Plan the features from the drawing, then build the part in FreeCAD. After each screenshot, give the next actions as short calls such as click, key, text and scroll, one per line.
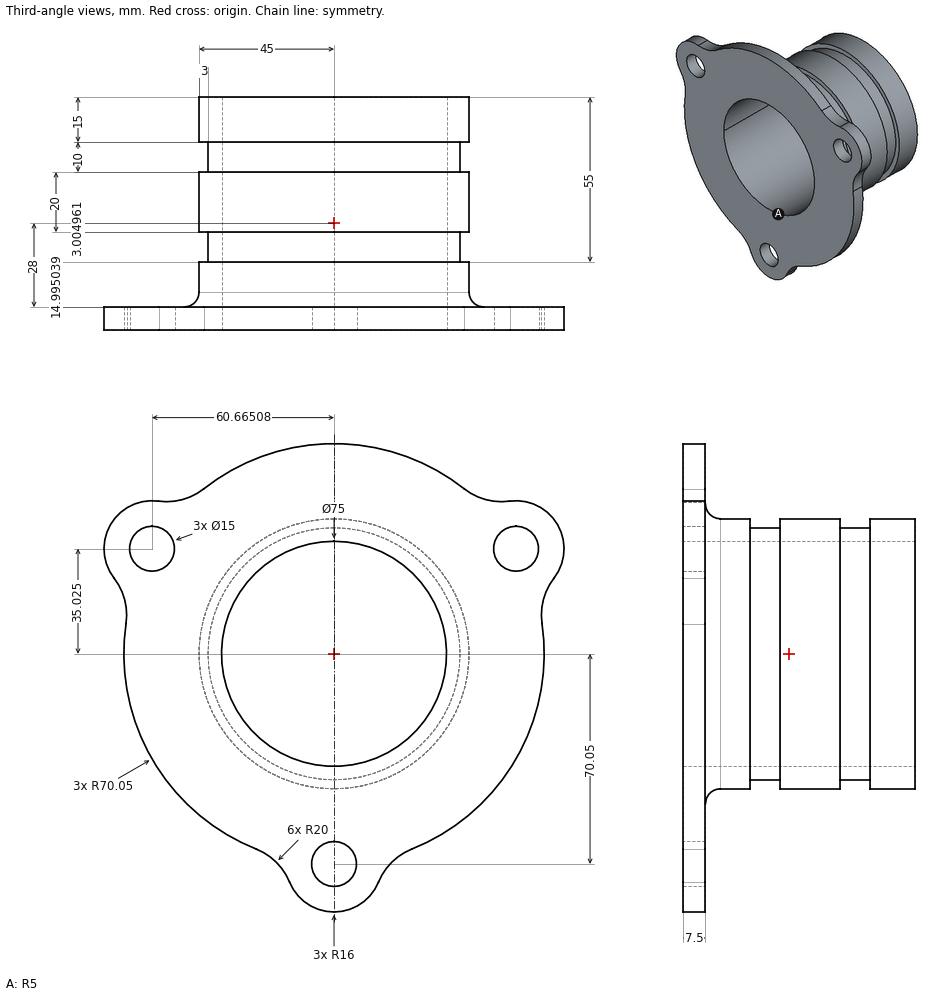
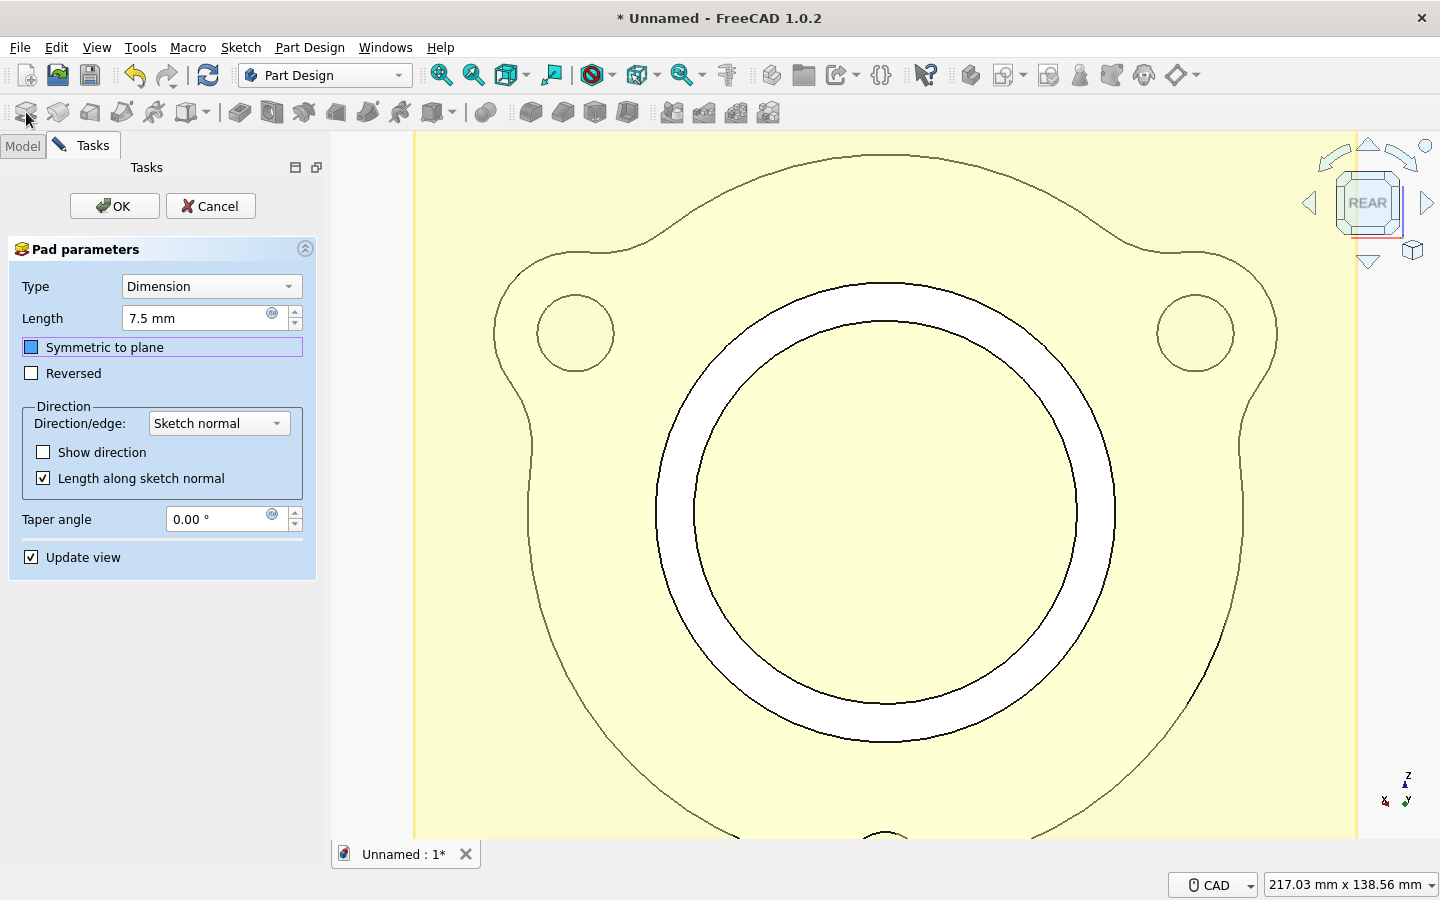
click(115, 206)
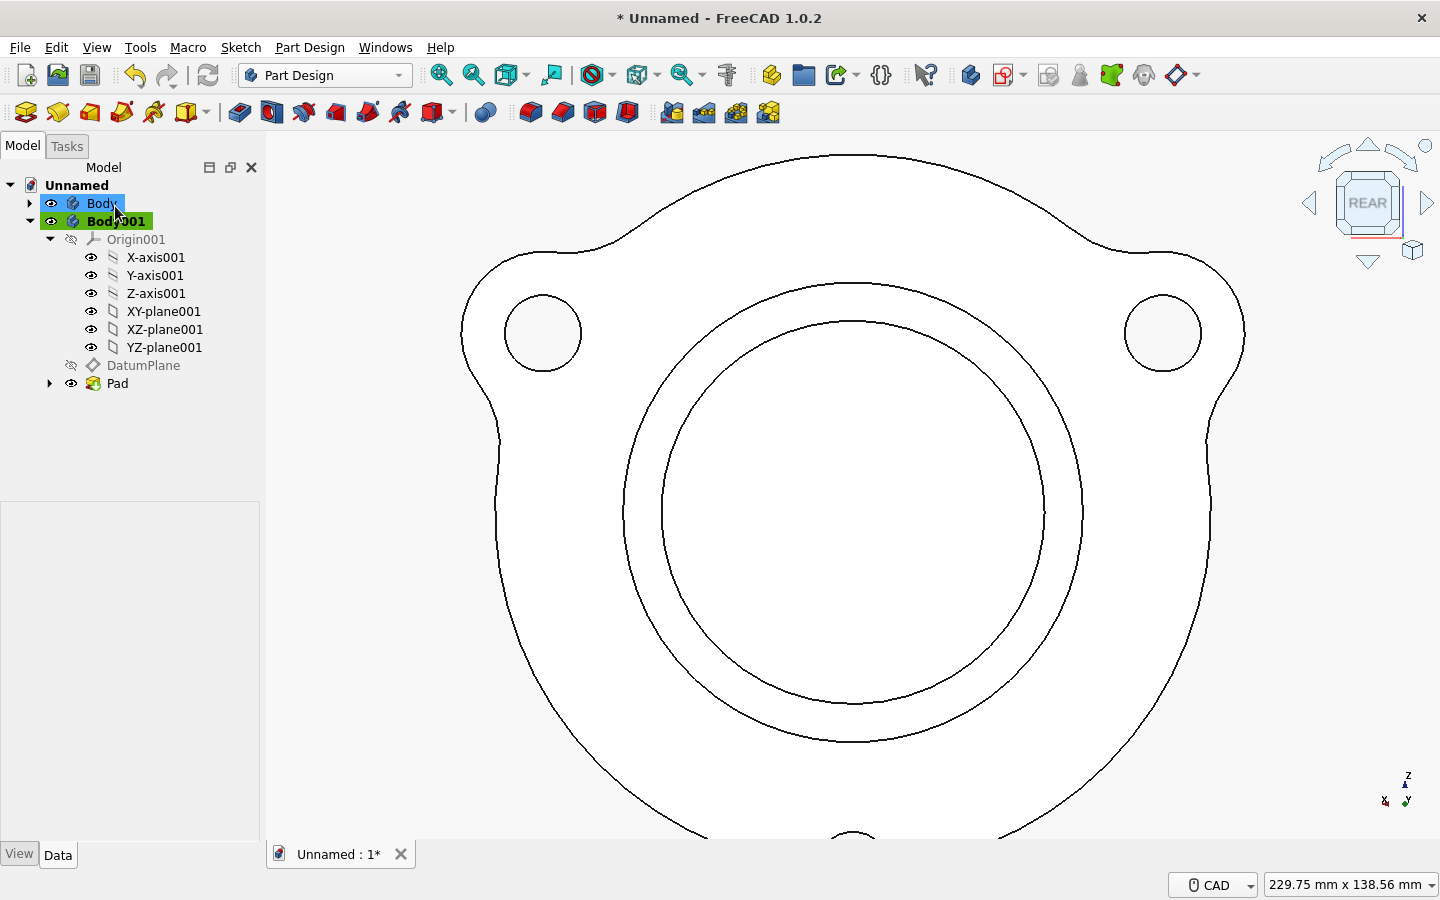
click(442, 76)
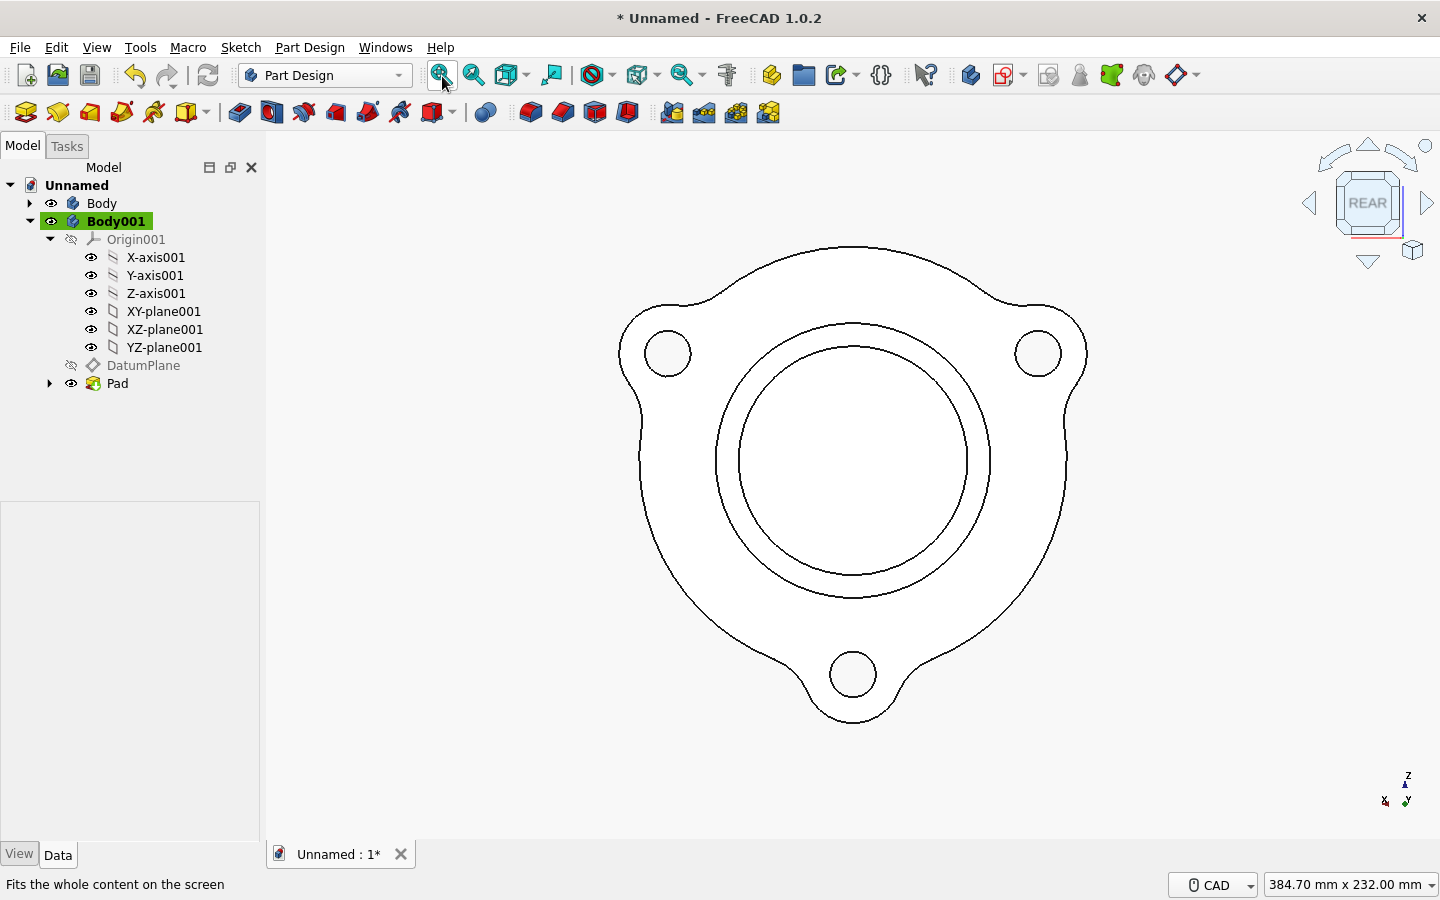
double_click(96, 203)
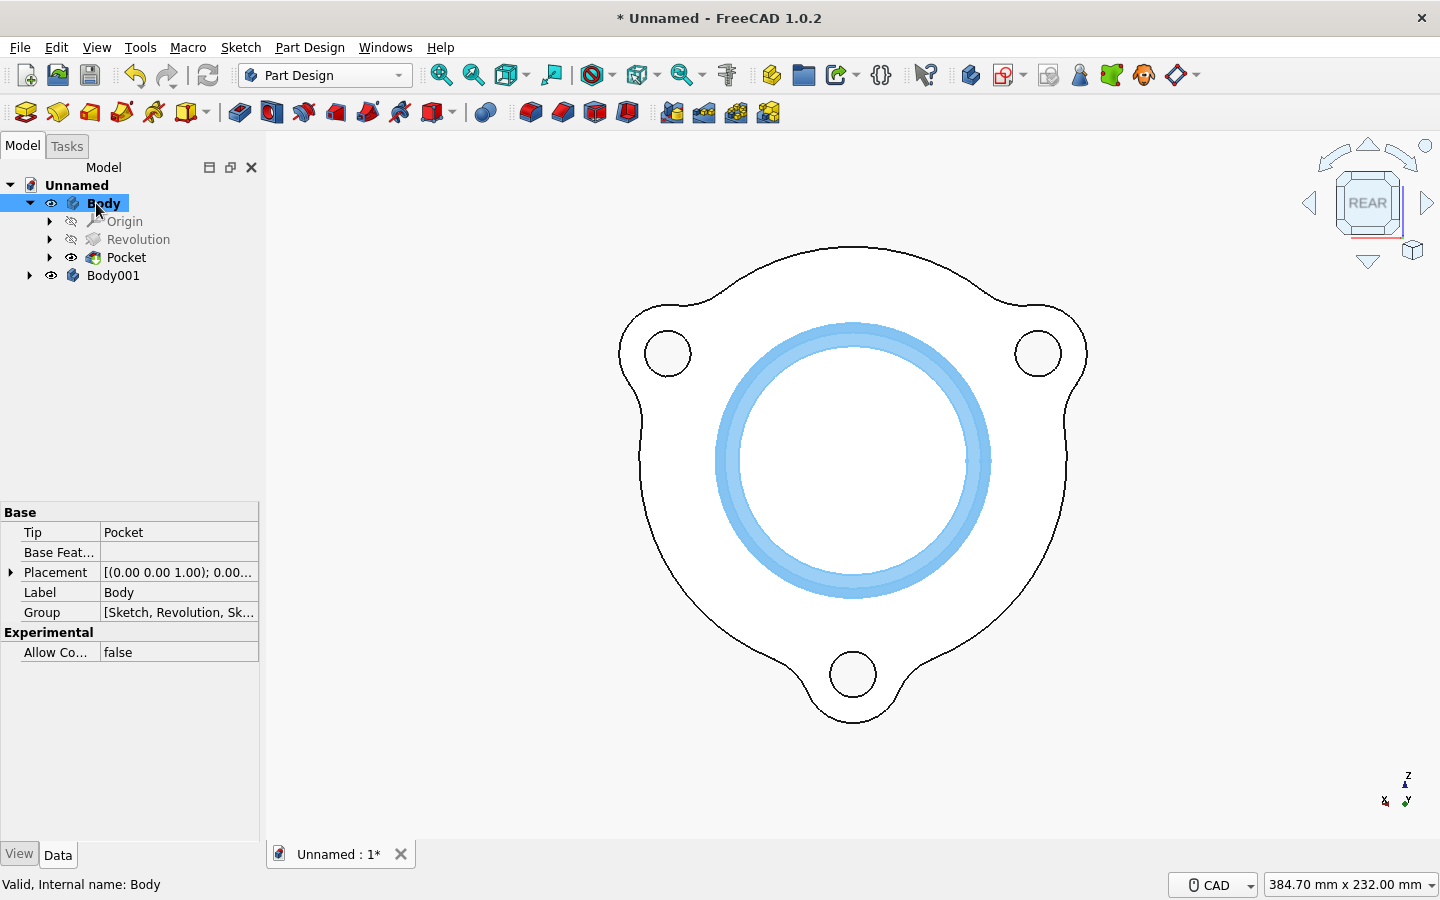
click(96, 203)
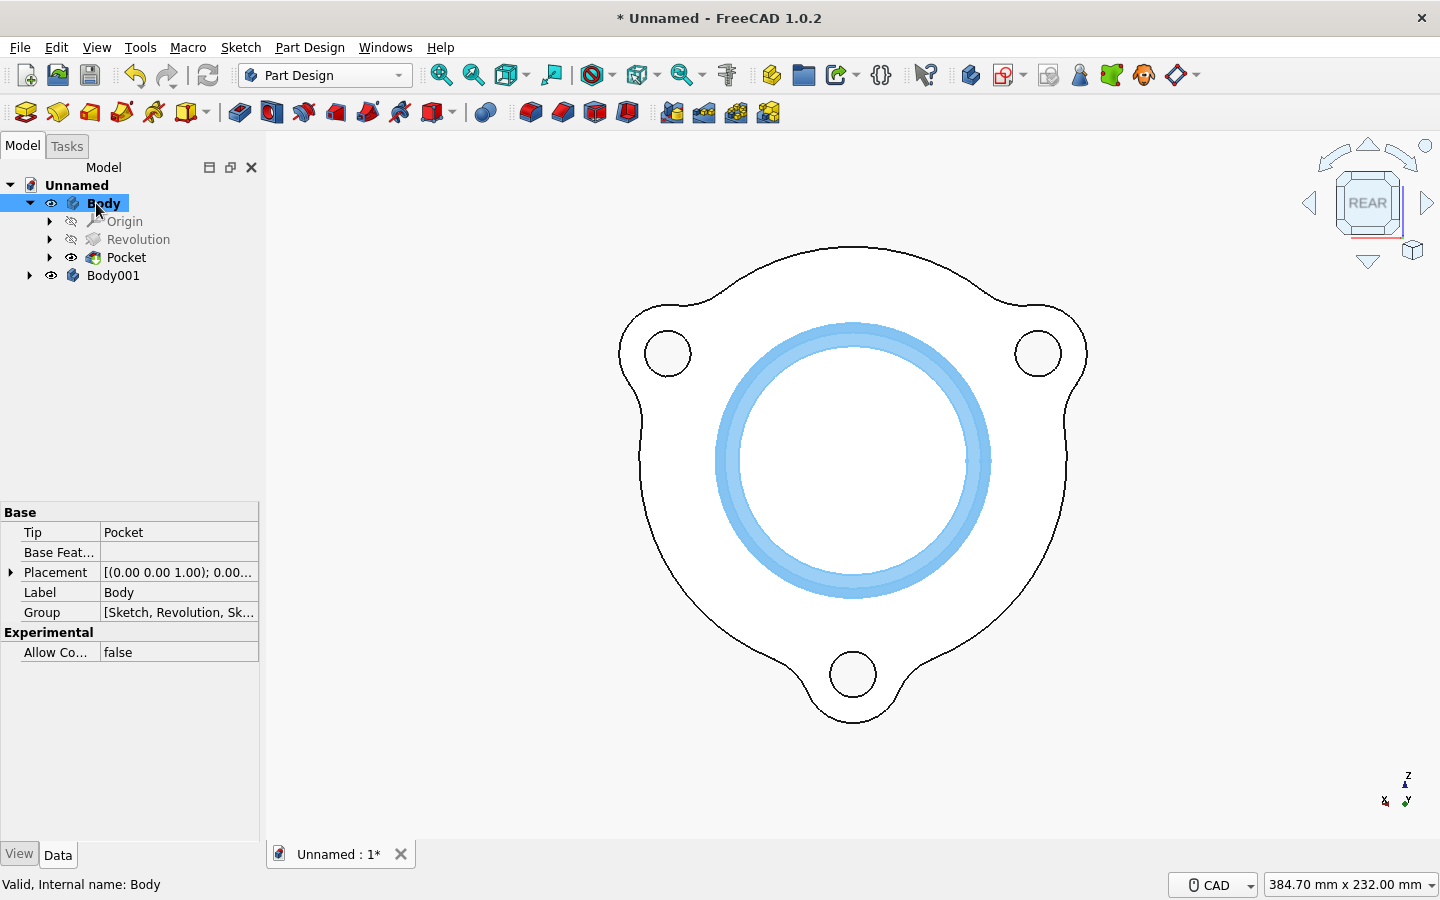
click(146, 652)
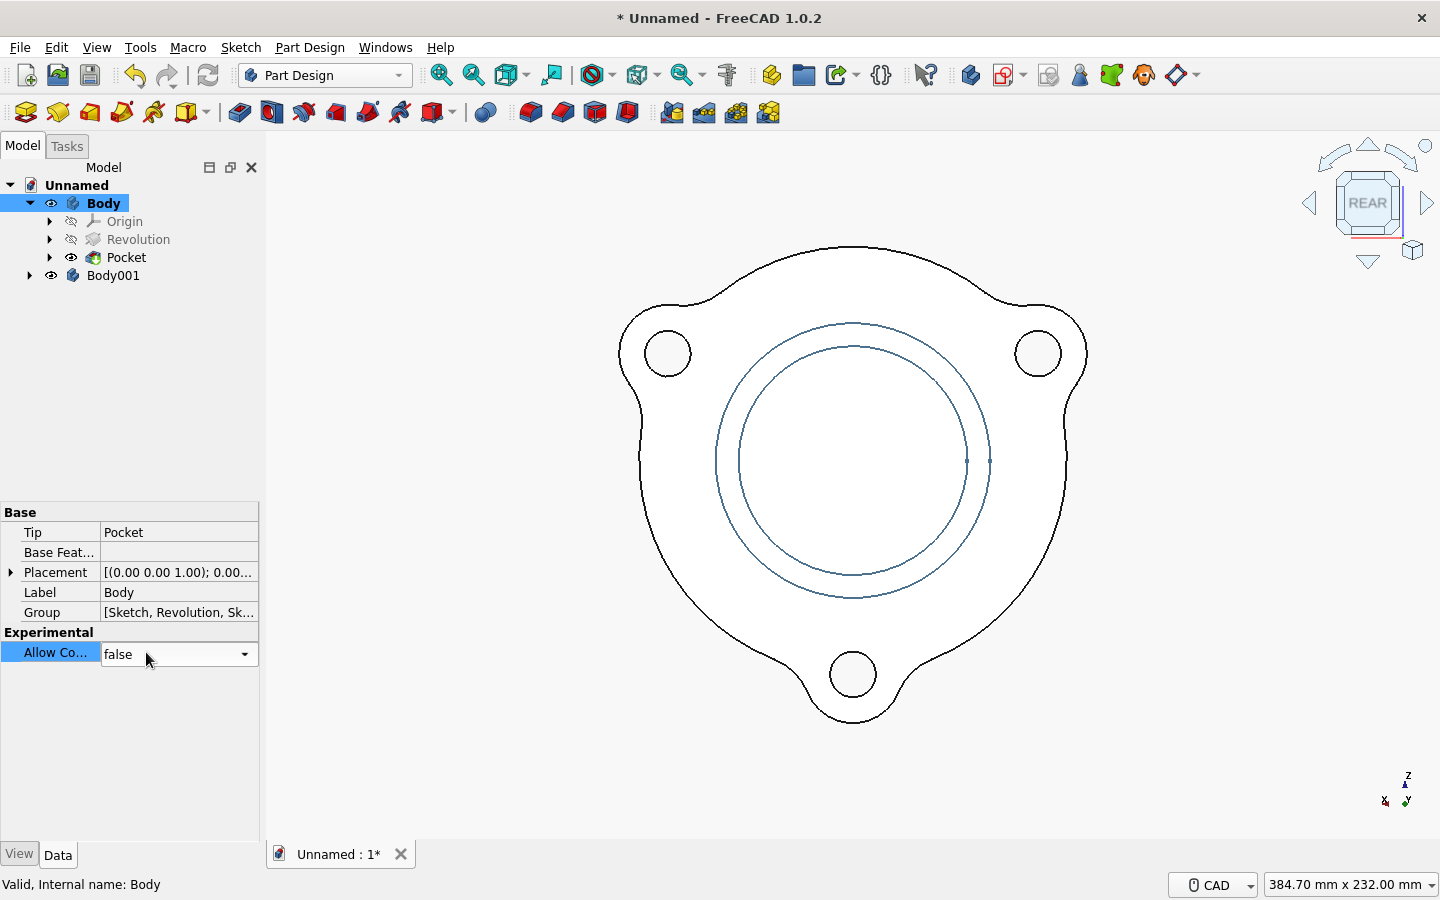
click(146, 652)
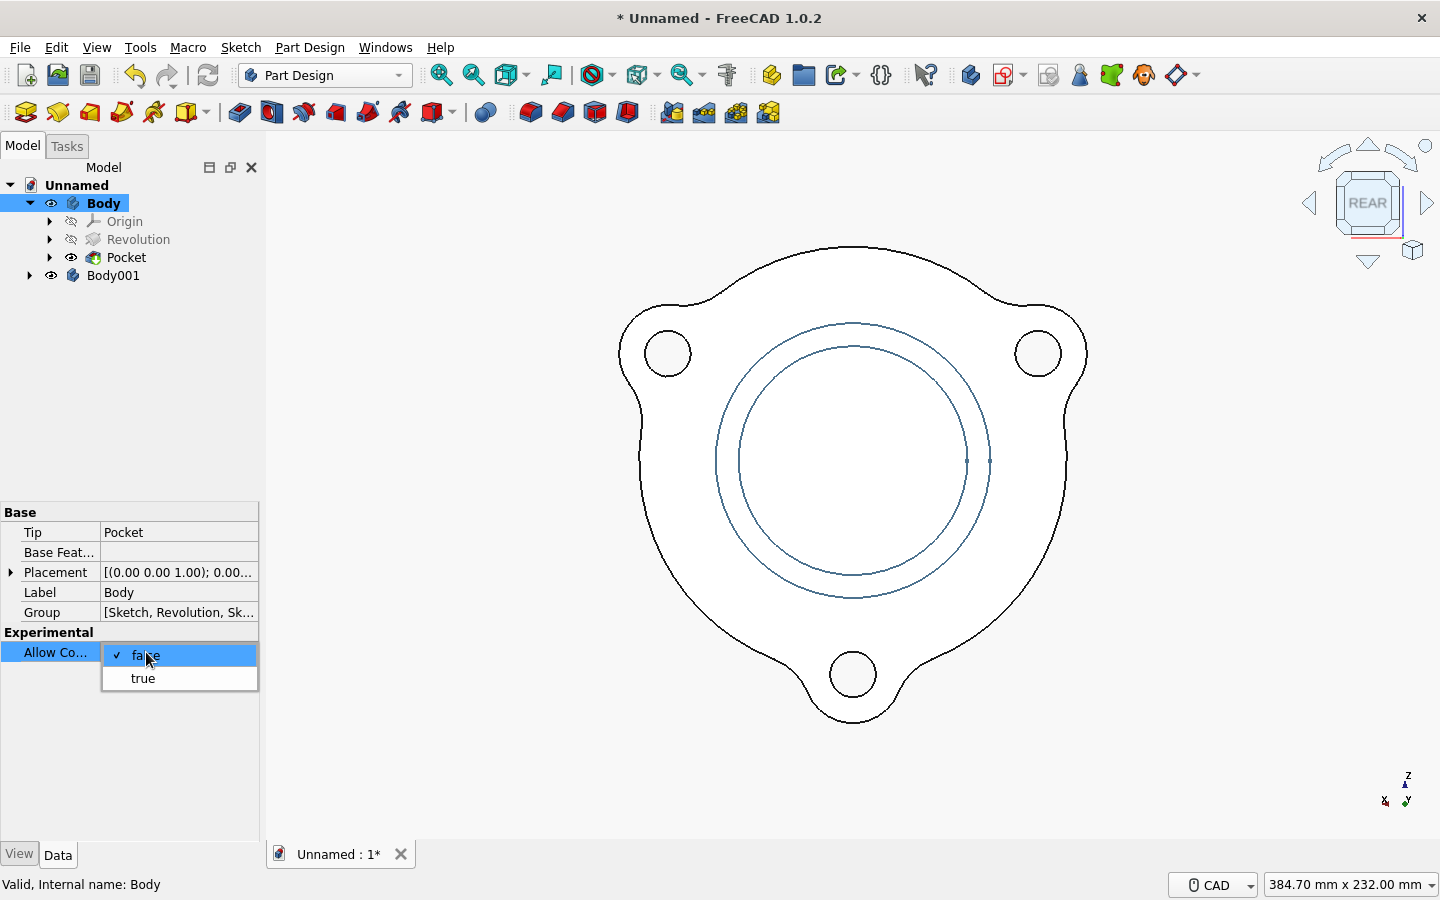
click(179, 678)
key(Return)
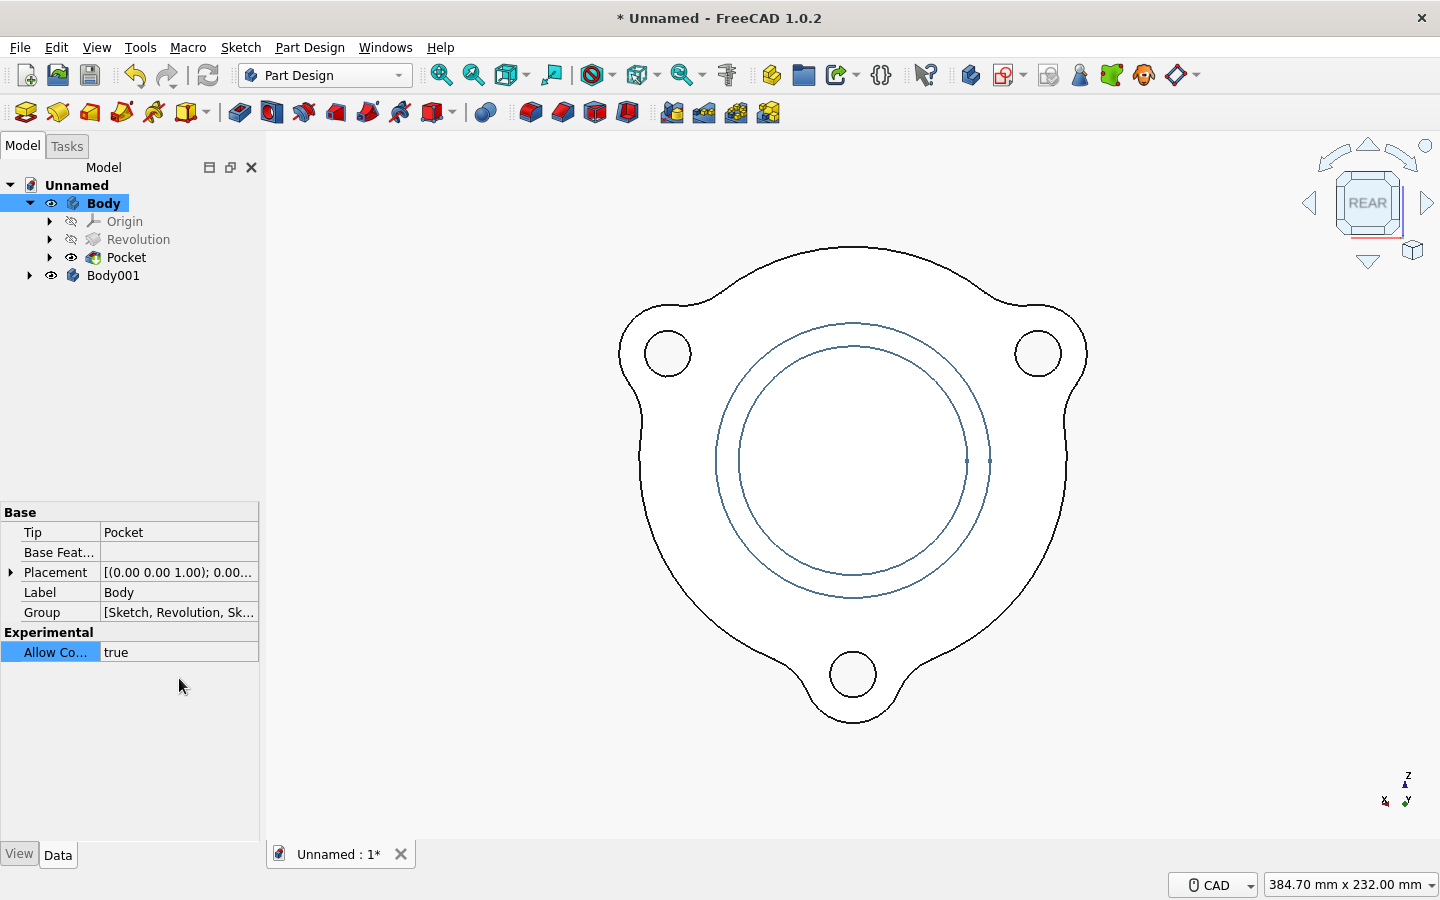
click(96, 275)